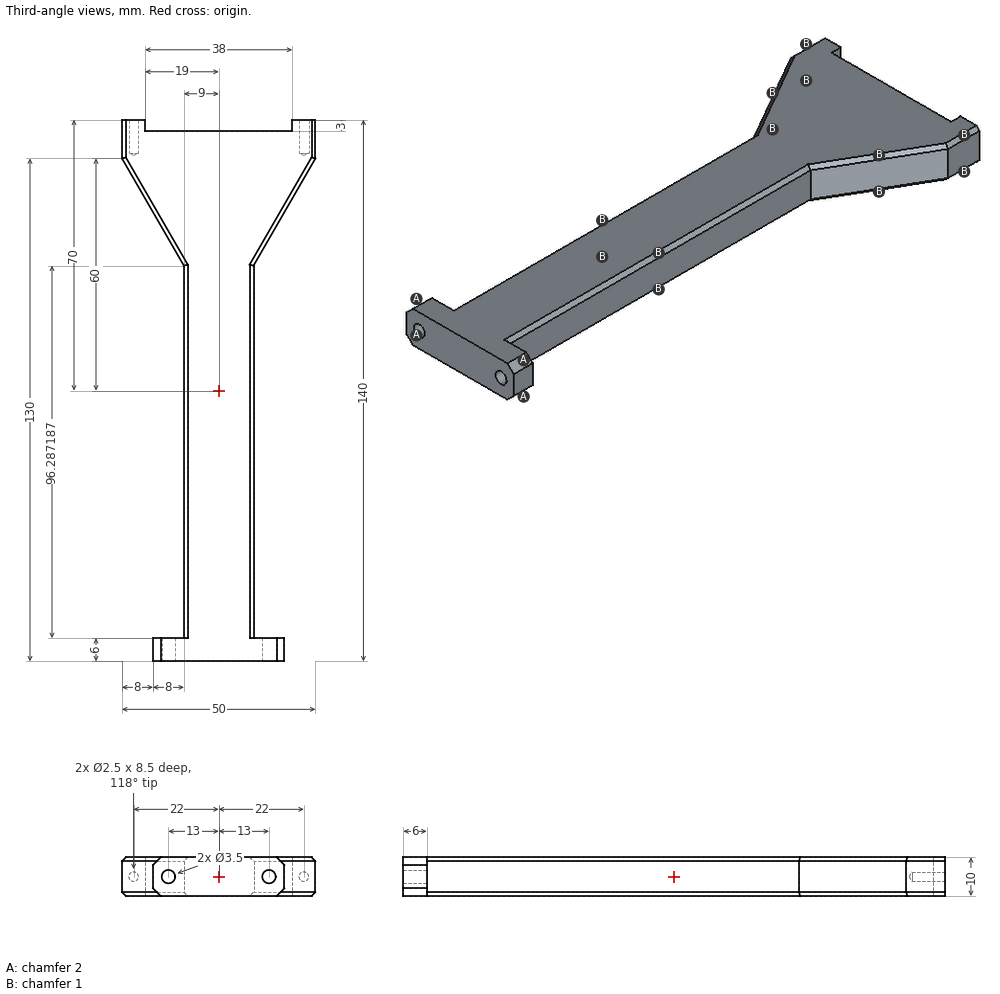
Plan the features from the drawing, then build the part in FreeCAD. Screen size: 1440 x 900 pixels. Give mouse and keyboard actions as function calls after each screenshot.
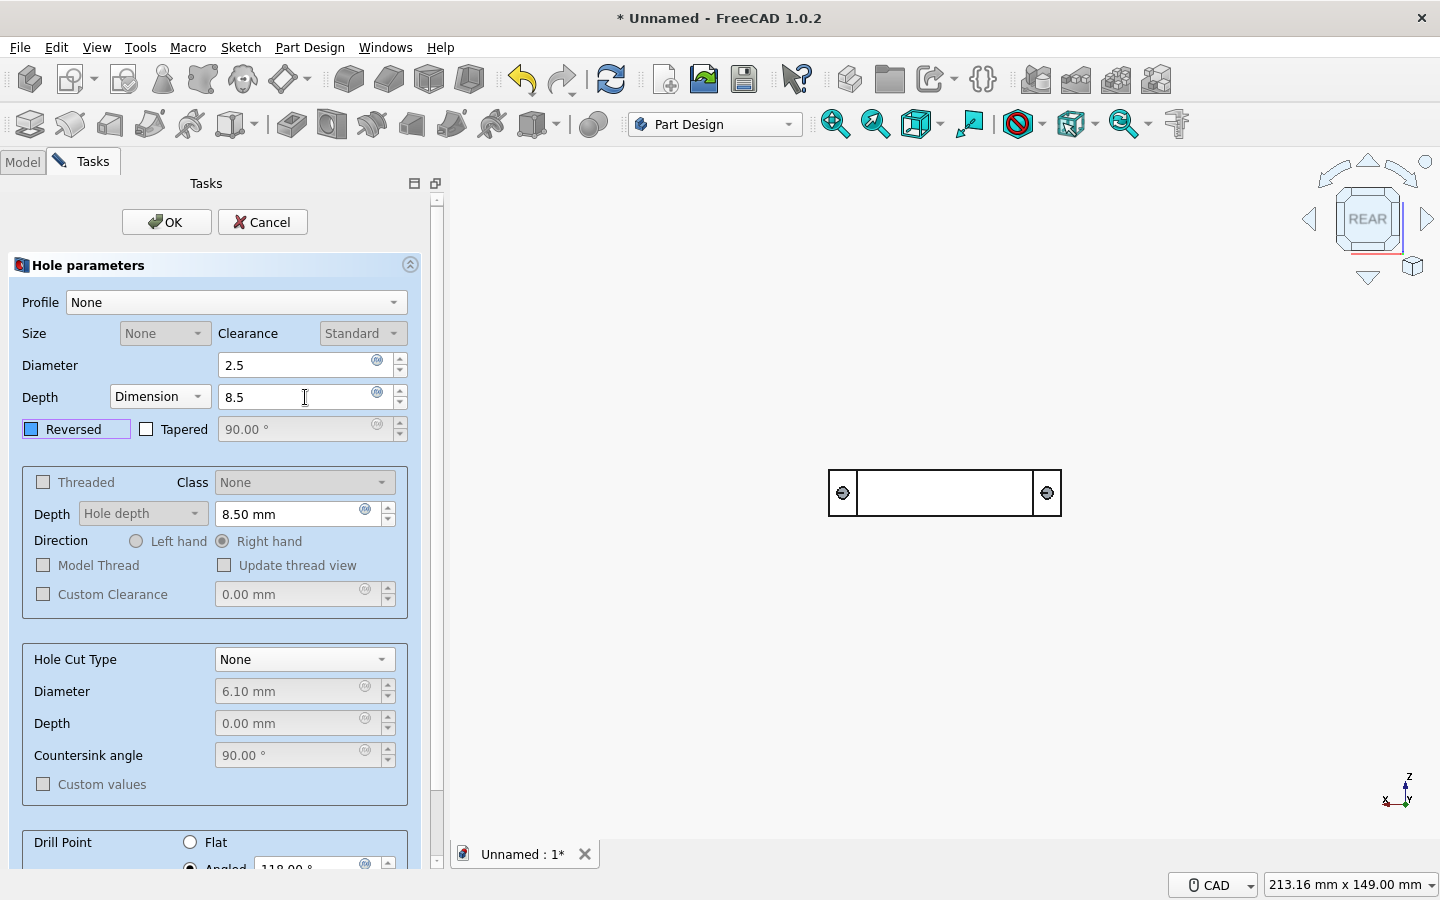
click(167, 222)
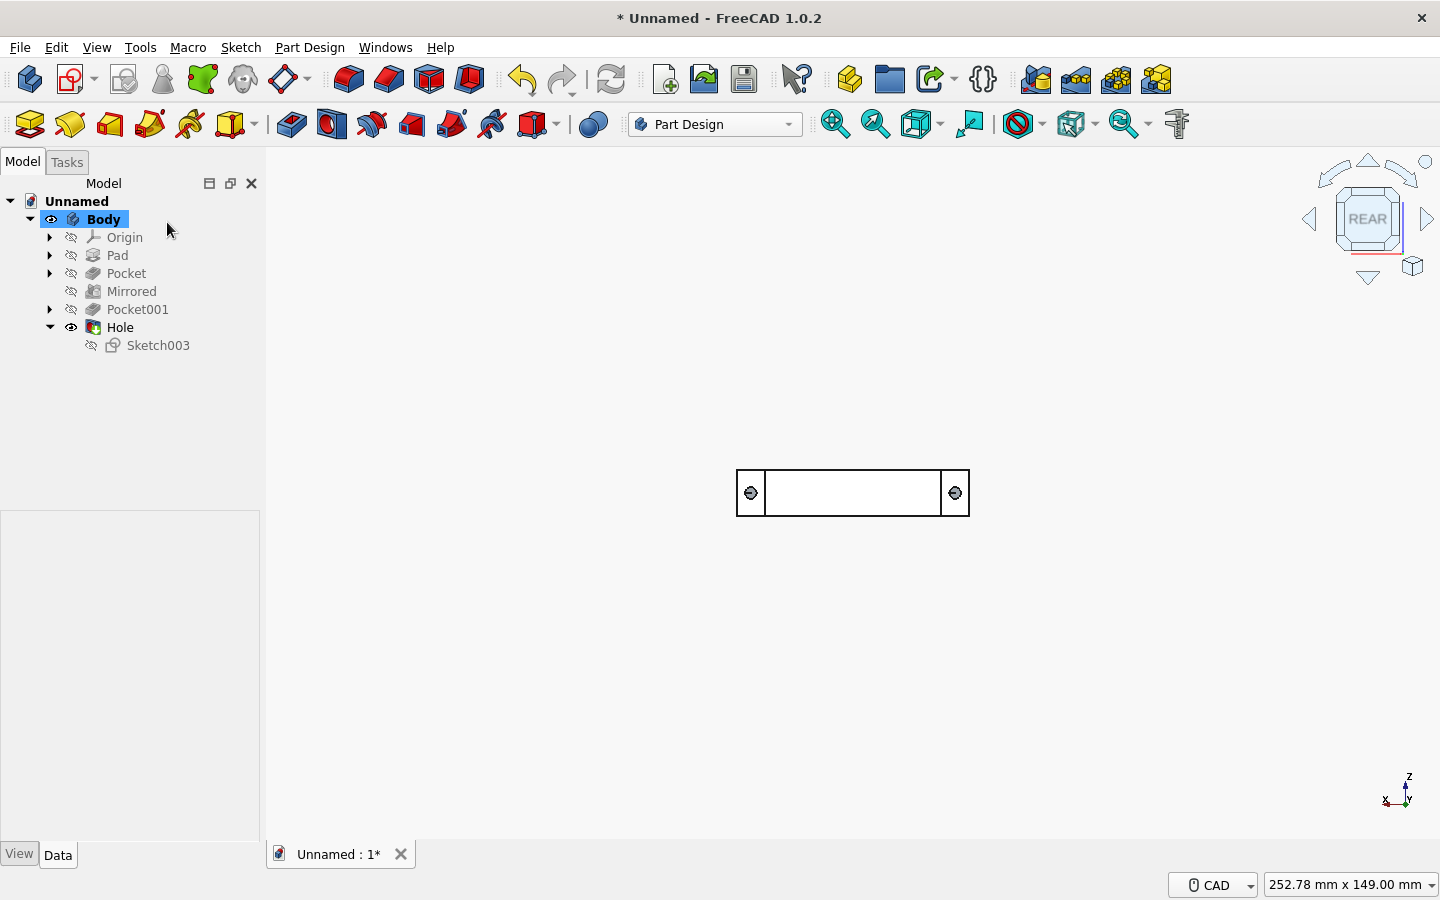
key(v)
key(f)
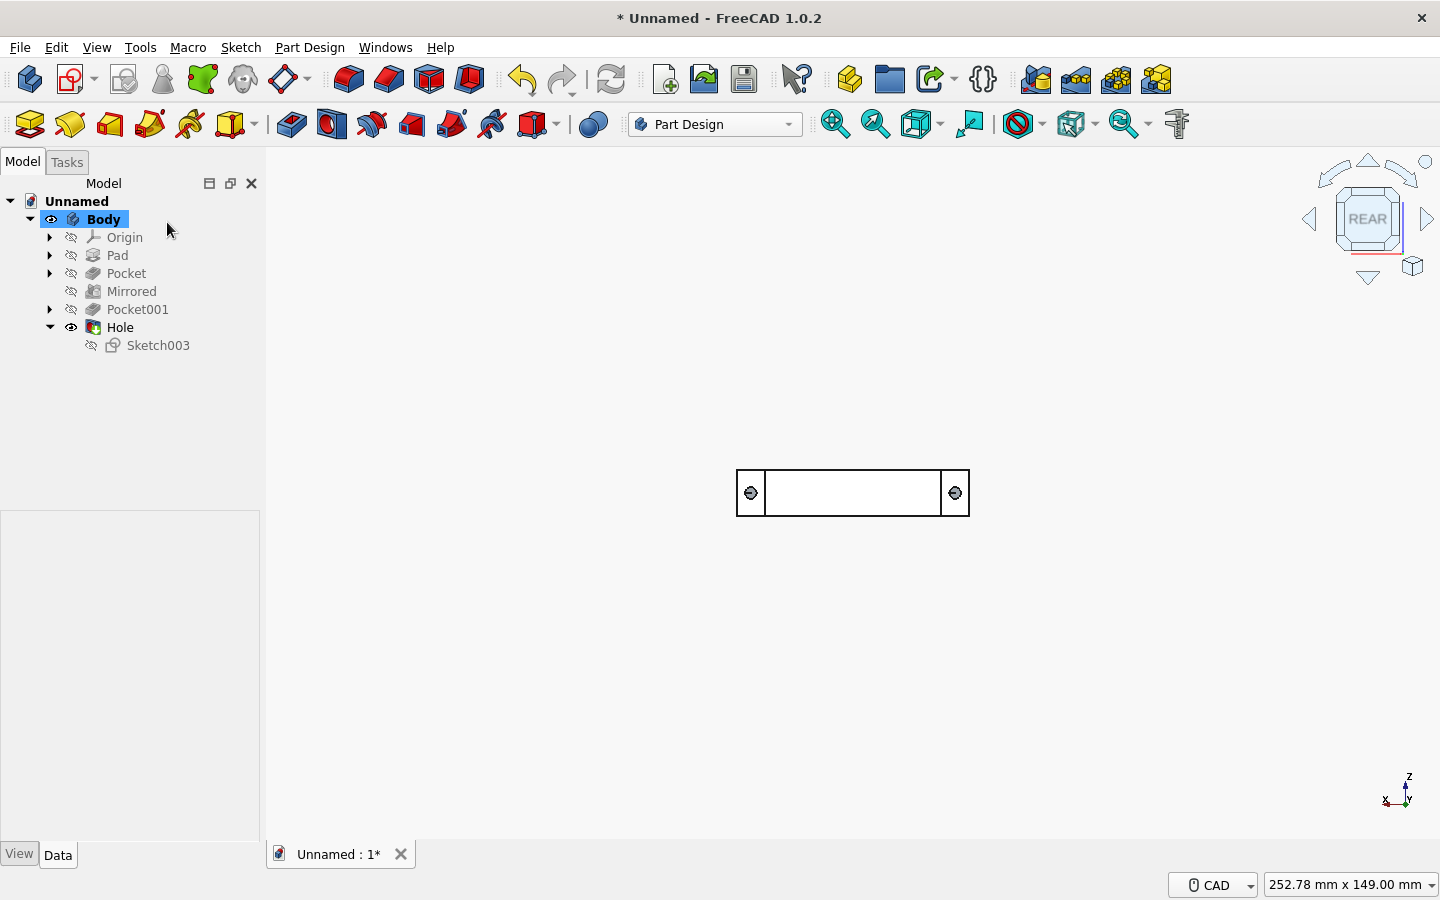
key(0)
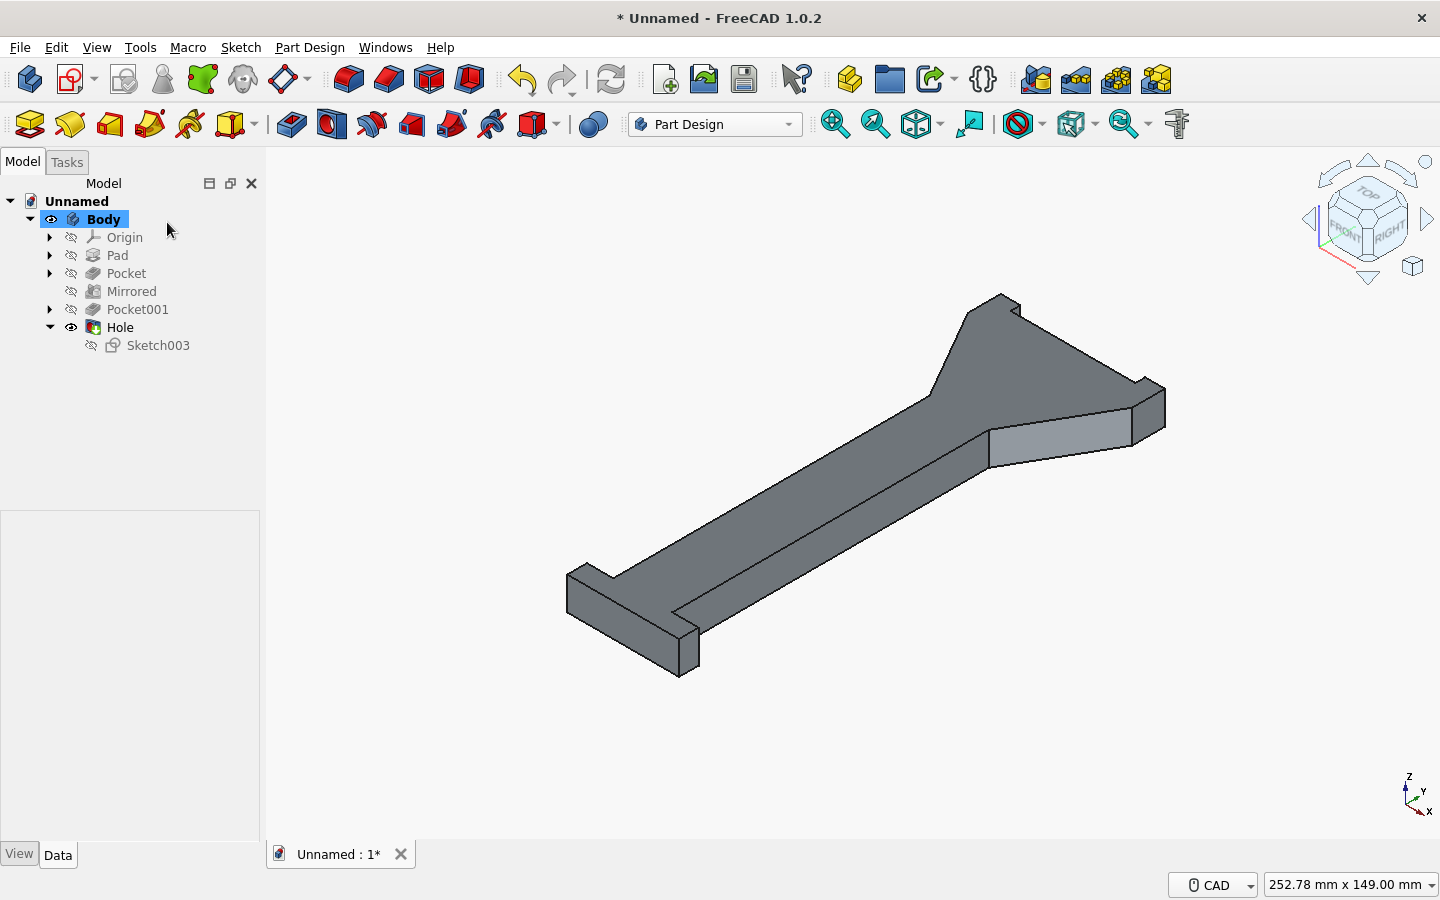
click(655, 643)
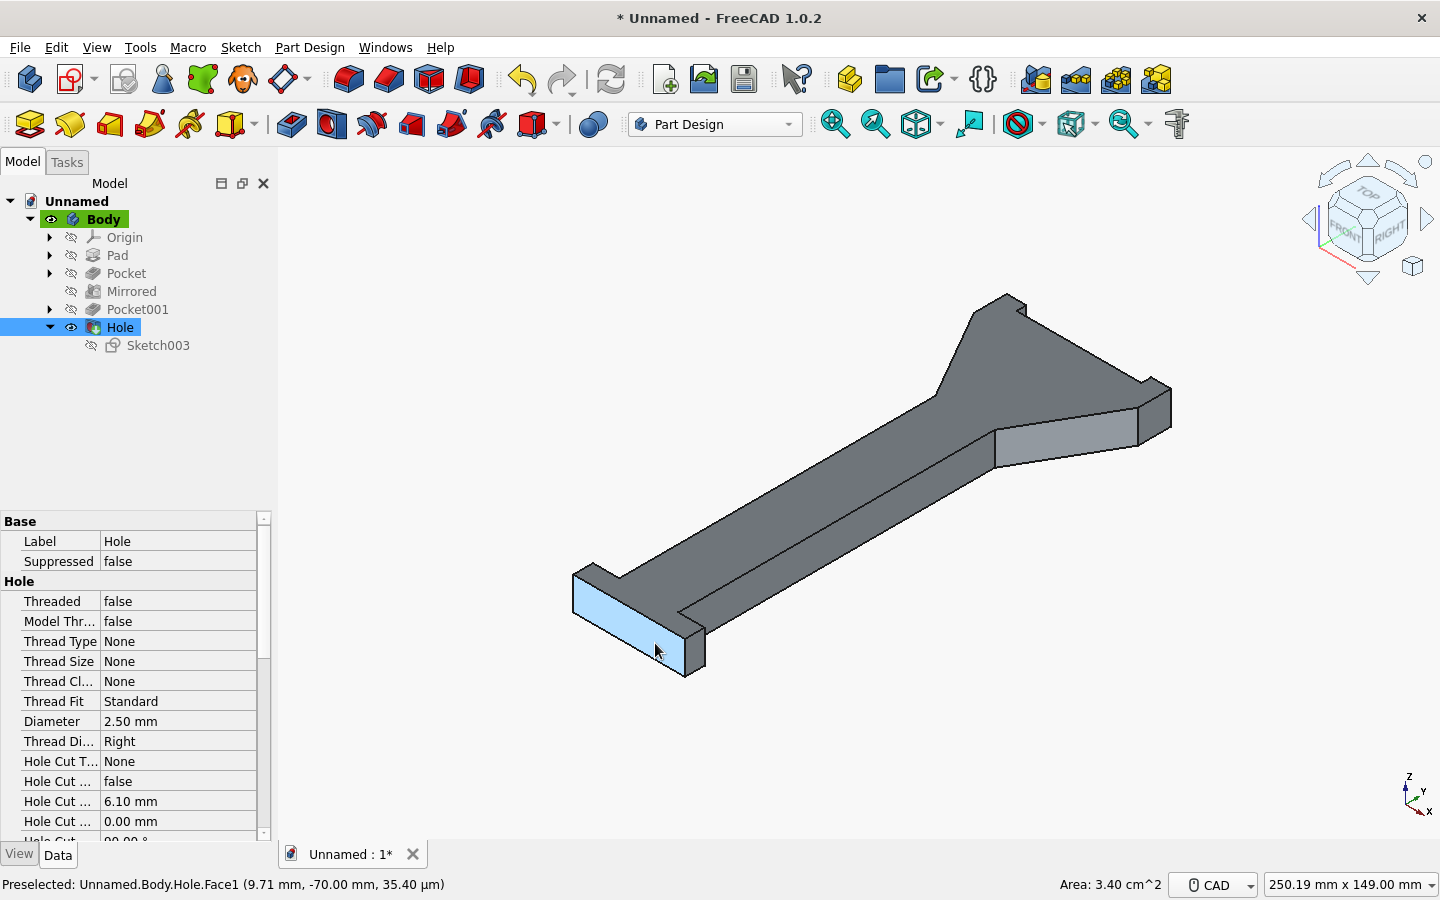
click(70, 80)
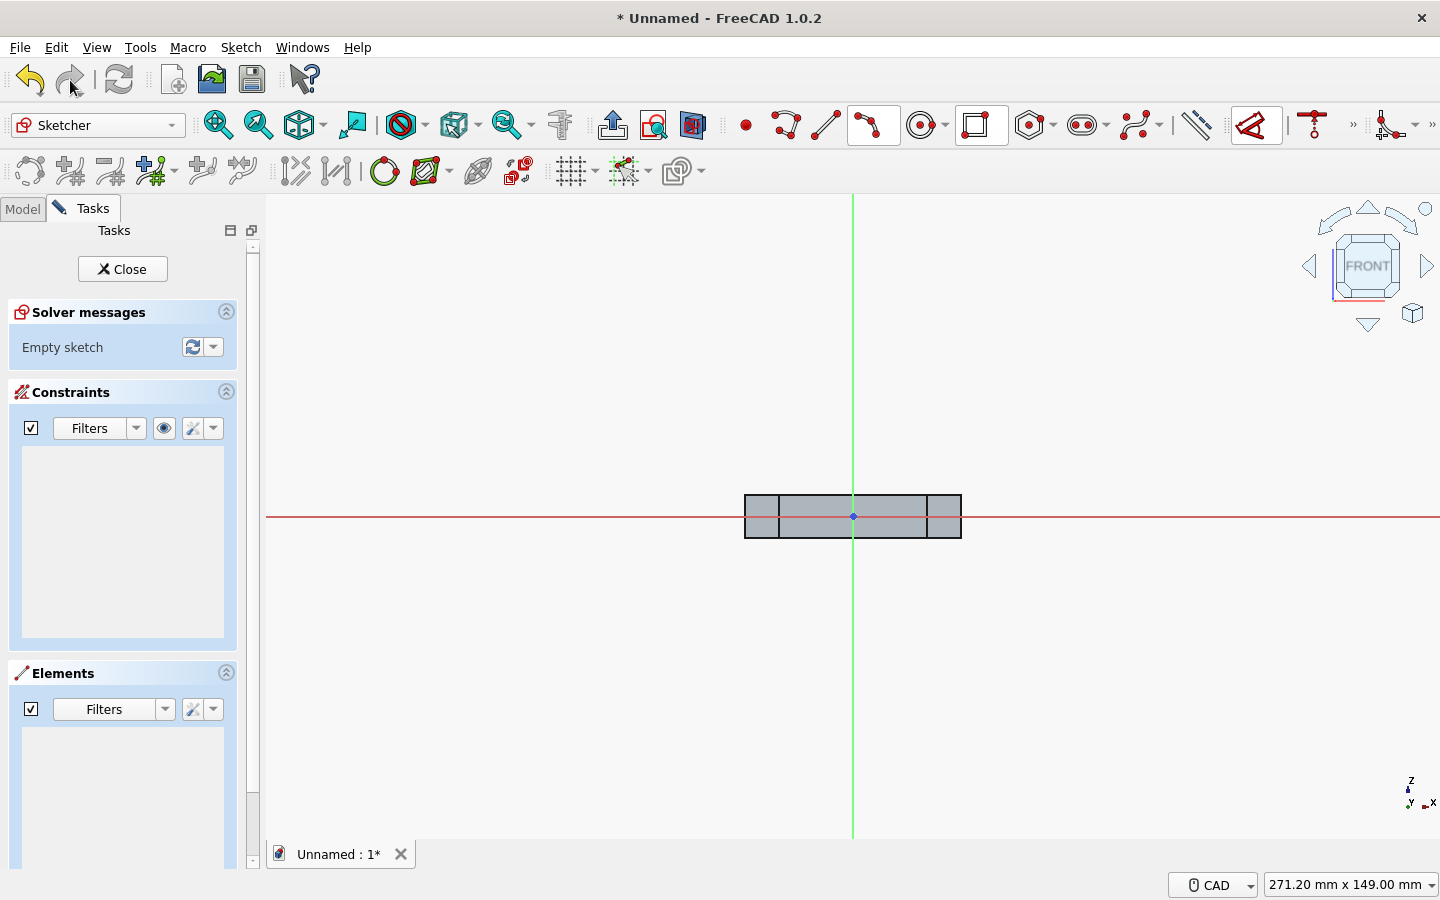
scroll(870, 516, up, 8)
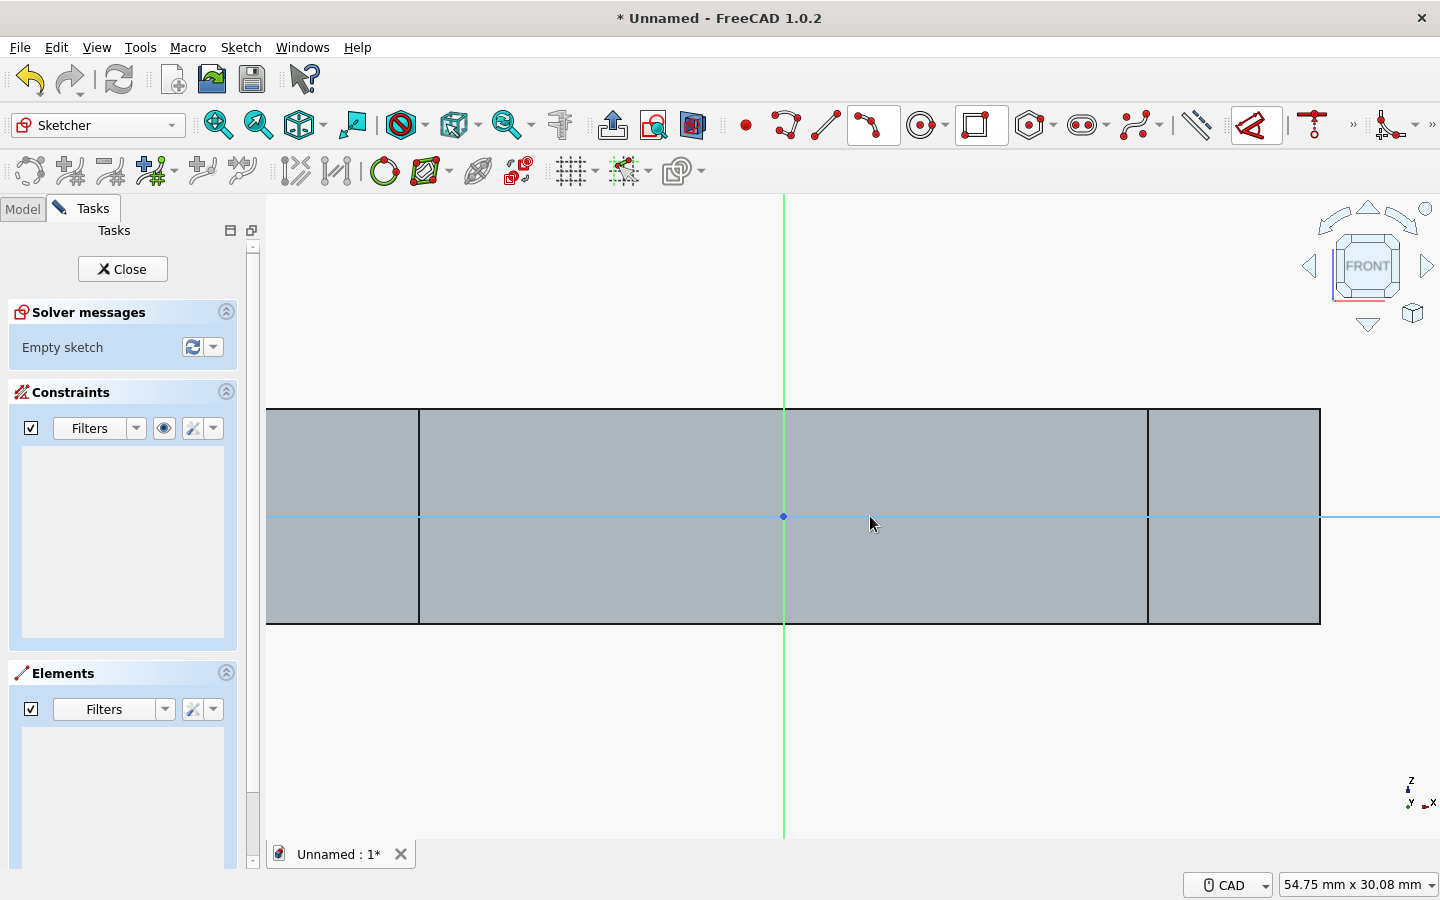
click(922, 126)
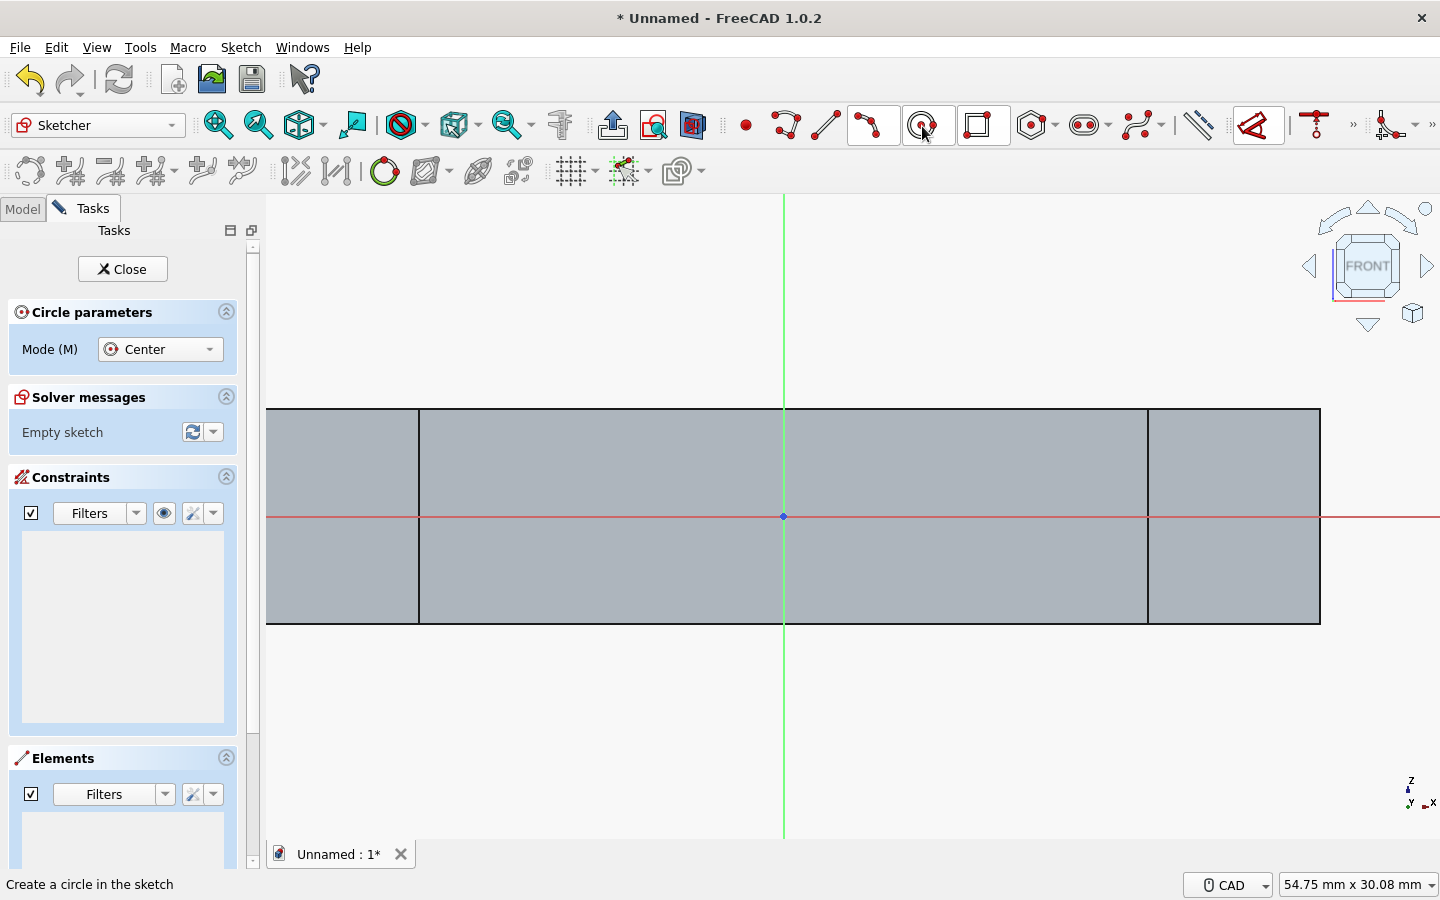
click(505, 516)
move(532, 490)